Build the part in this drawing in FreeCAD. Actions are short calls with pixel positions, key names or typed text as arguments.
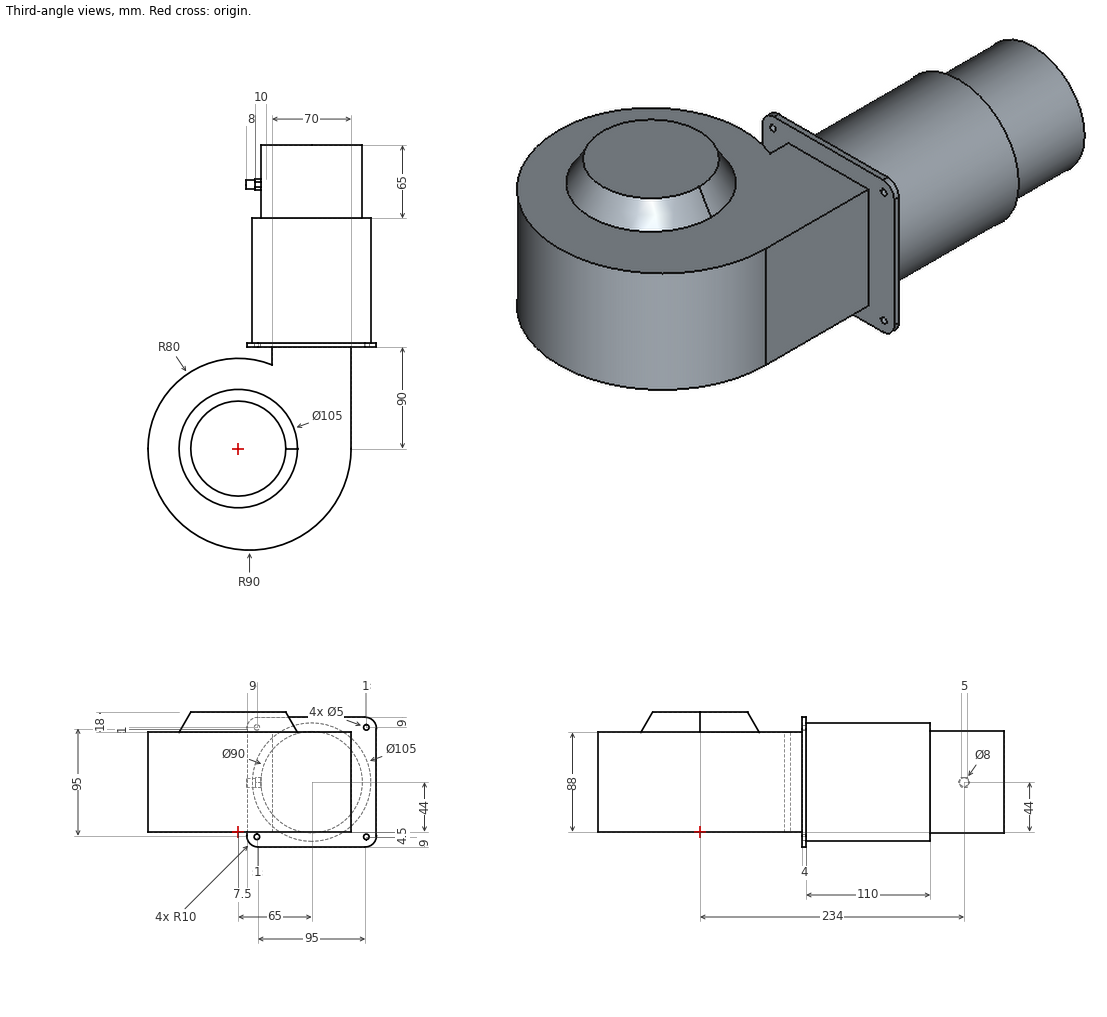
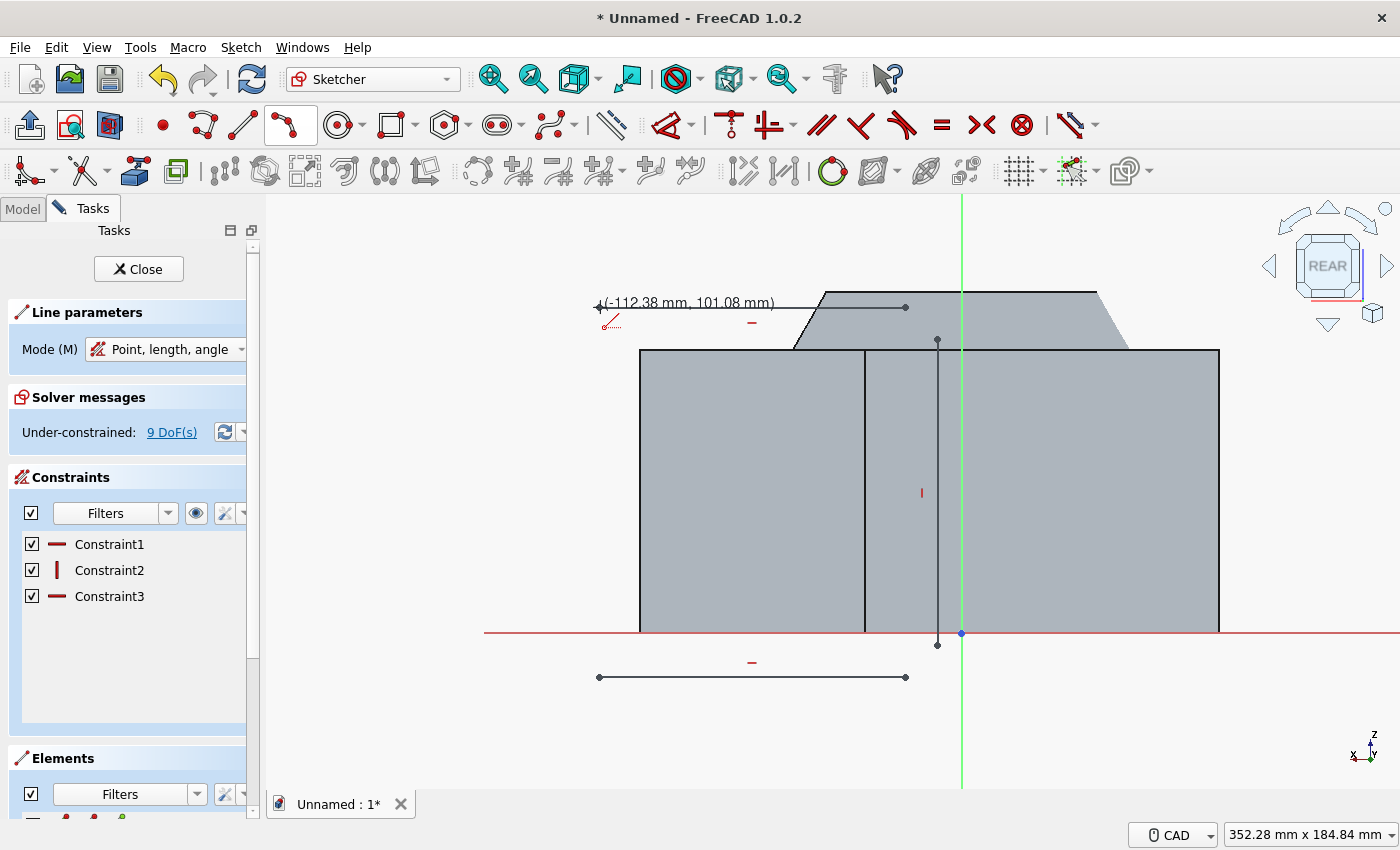
click(567, 339)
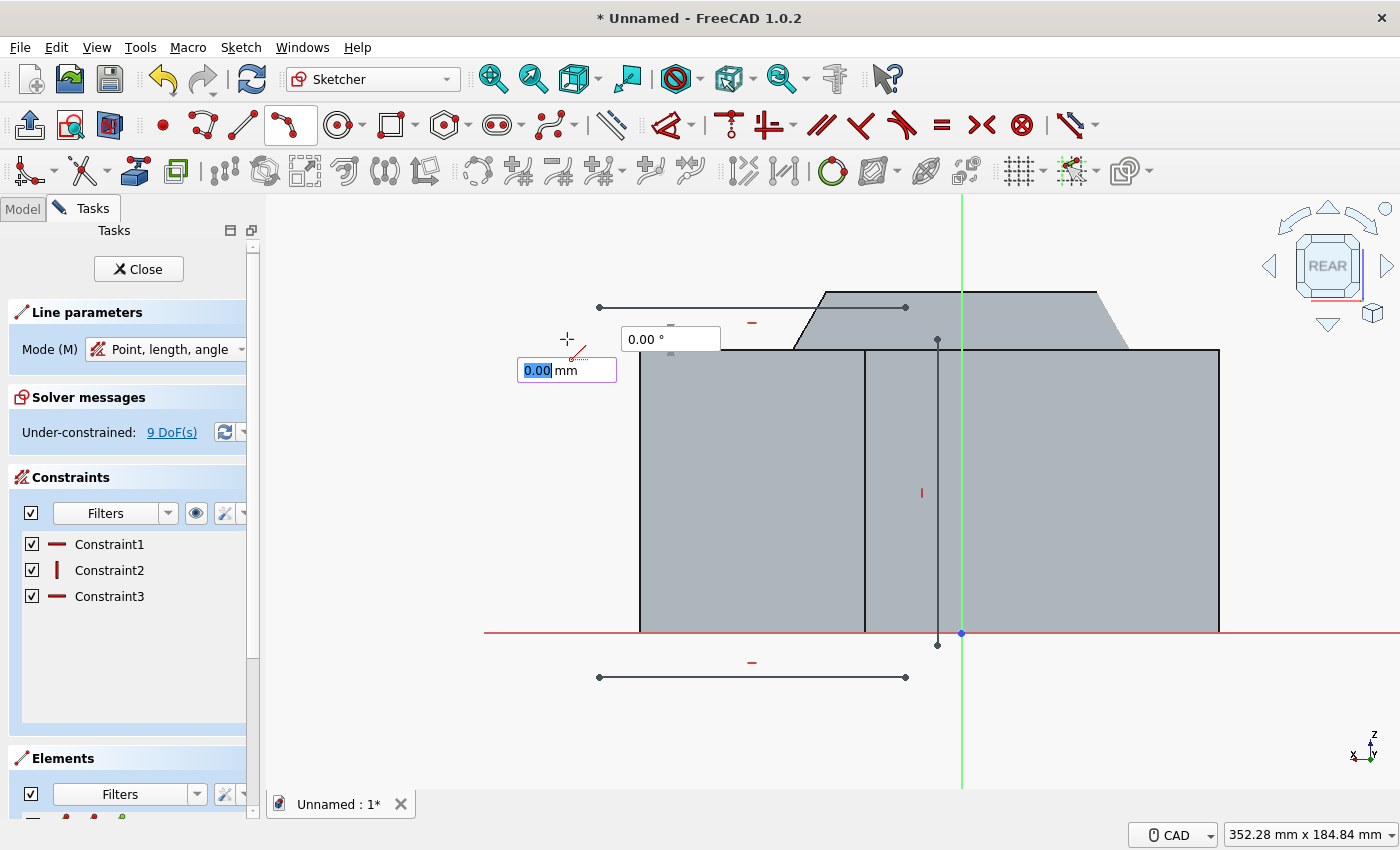
scroll(567, 645, up, 2)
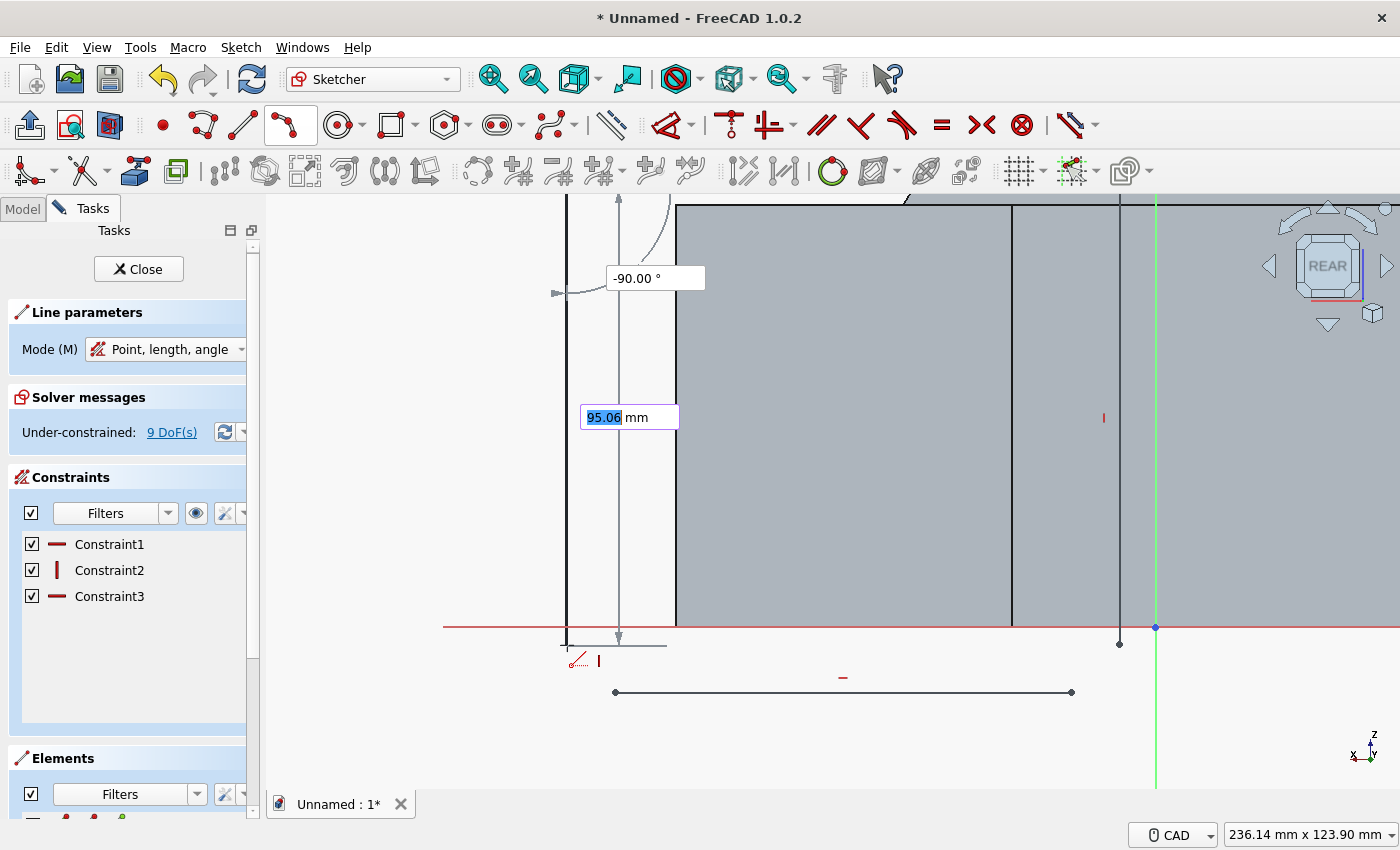
click(567, 644)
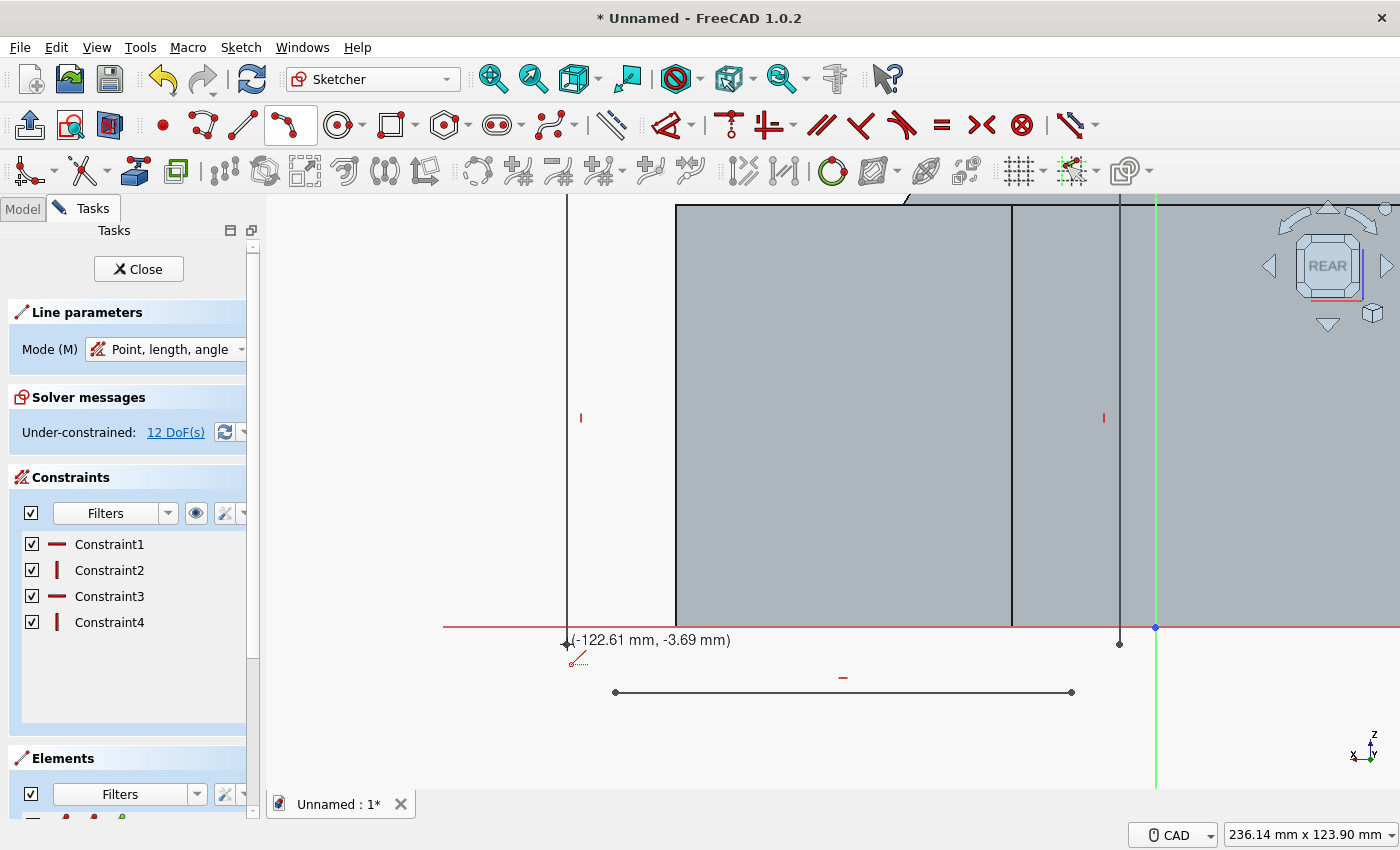
click(284, 126)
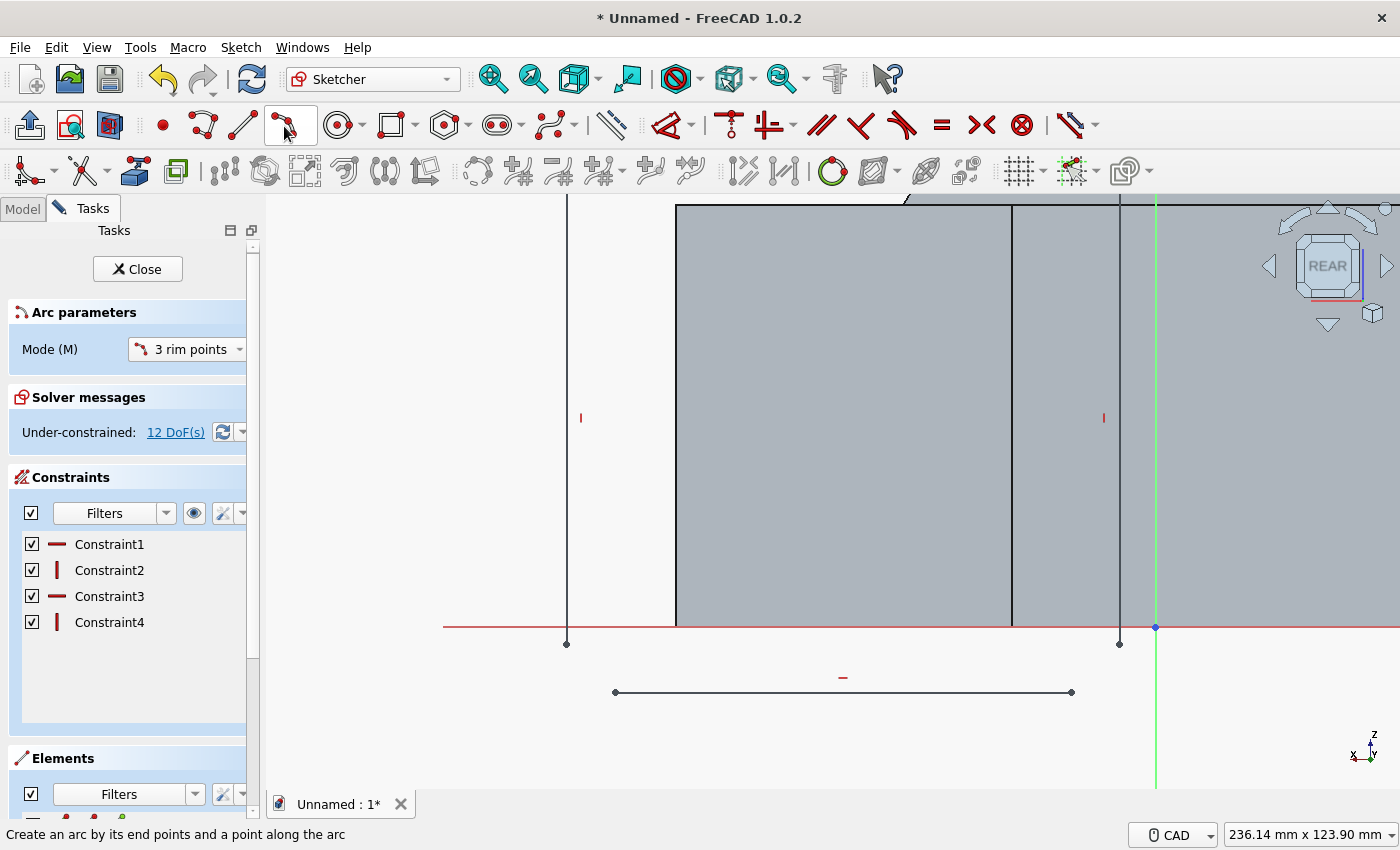
click(1072, 693)
click(1120, 645)
click(1106, 678)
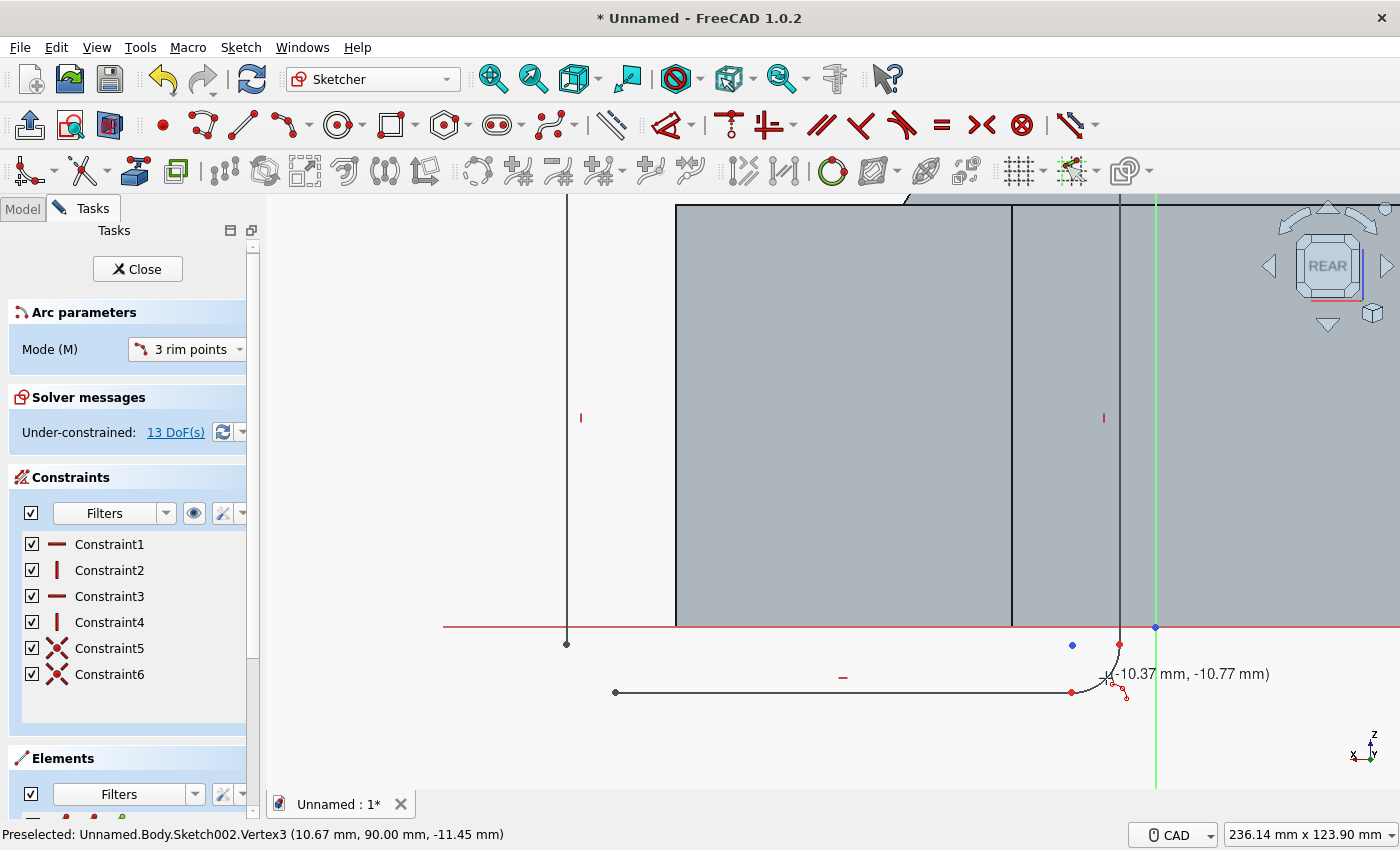
scroll(567, 645, down, 2)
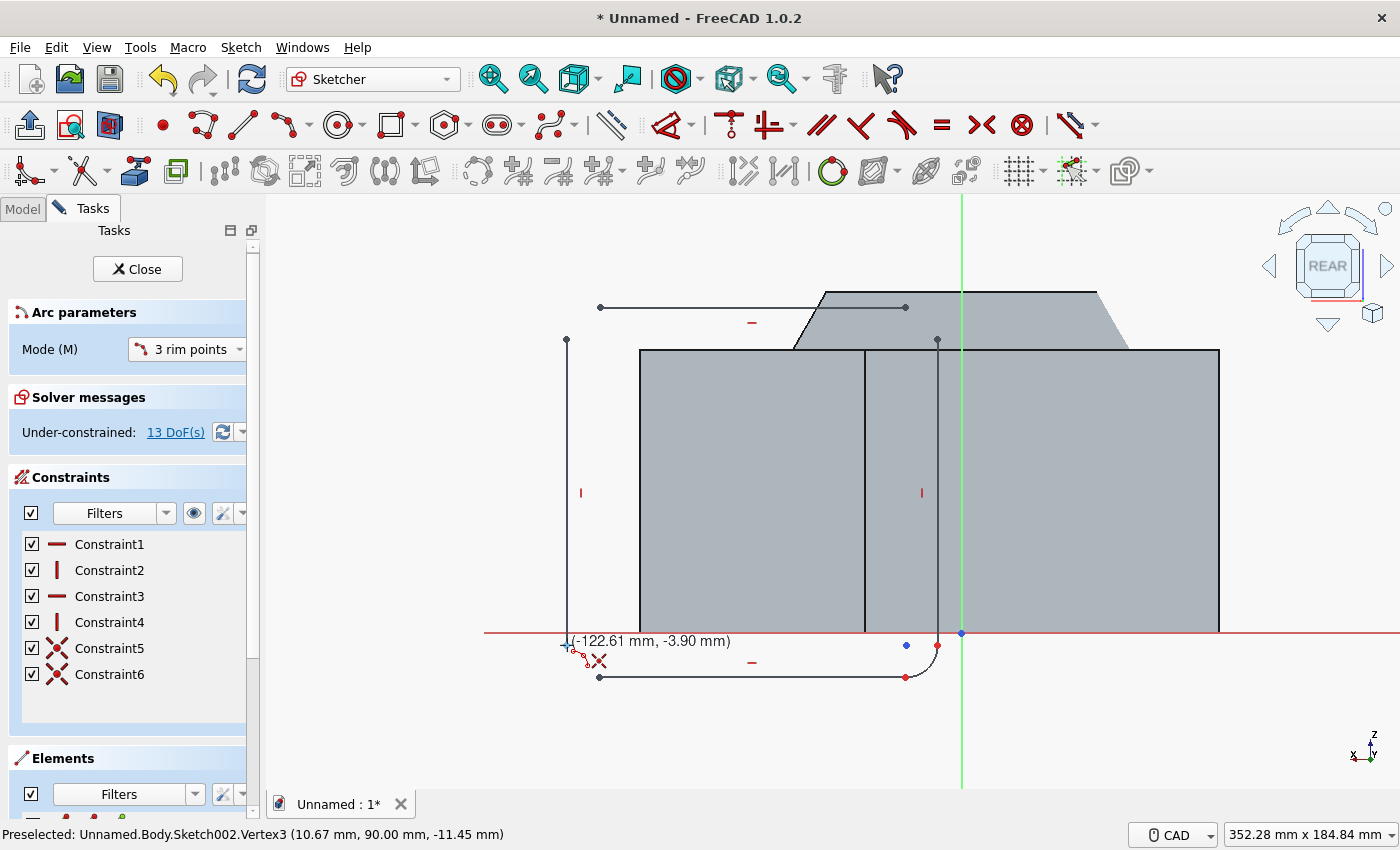
click(938, 340)
click(905, 308)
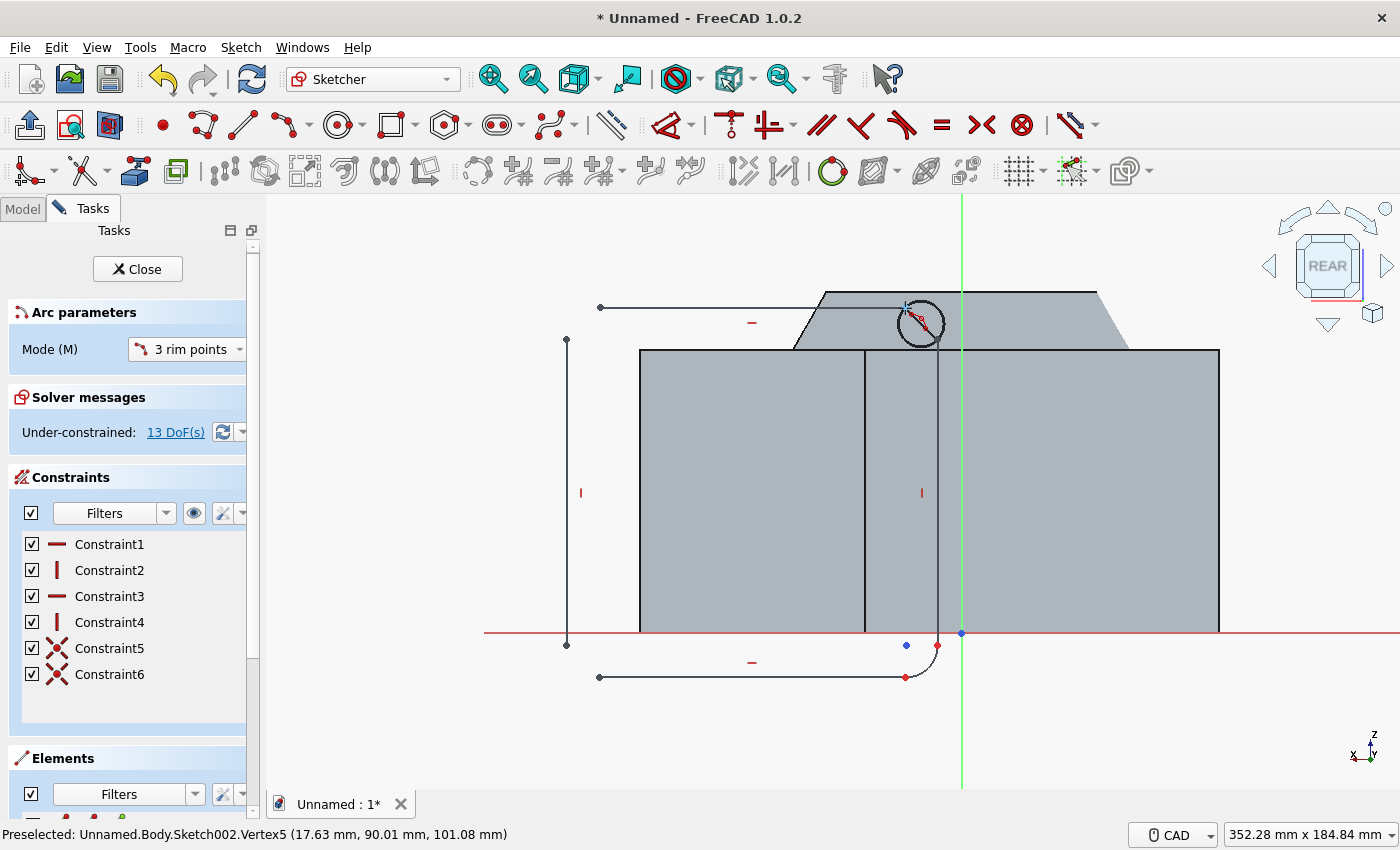
scroll(928, 316, up, 3)